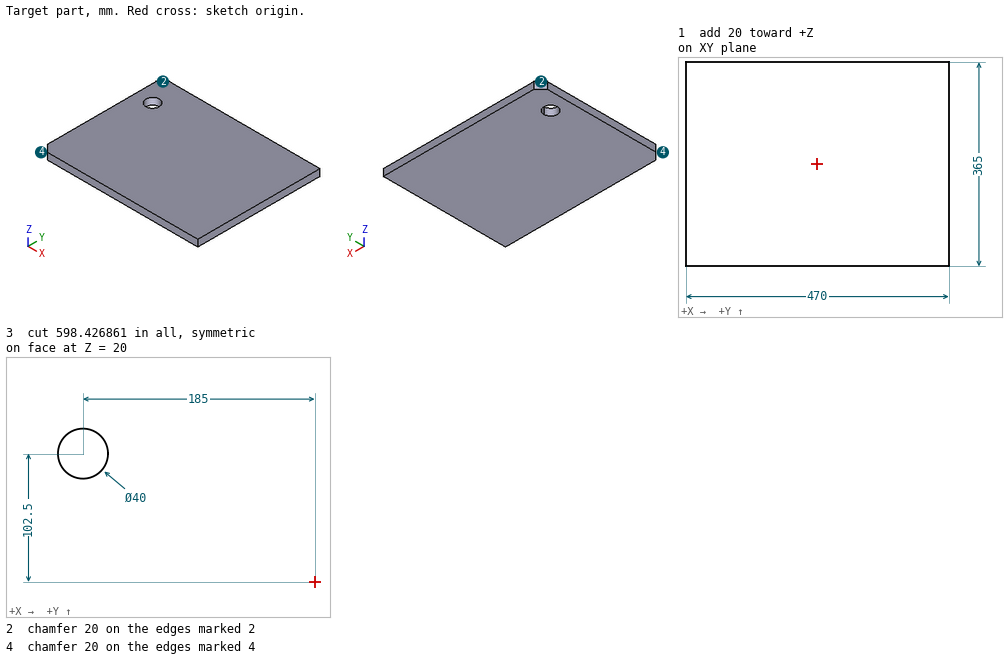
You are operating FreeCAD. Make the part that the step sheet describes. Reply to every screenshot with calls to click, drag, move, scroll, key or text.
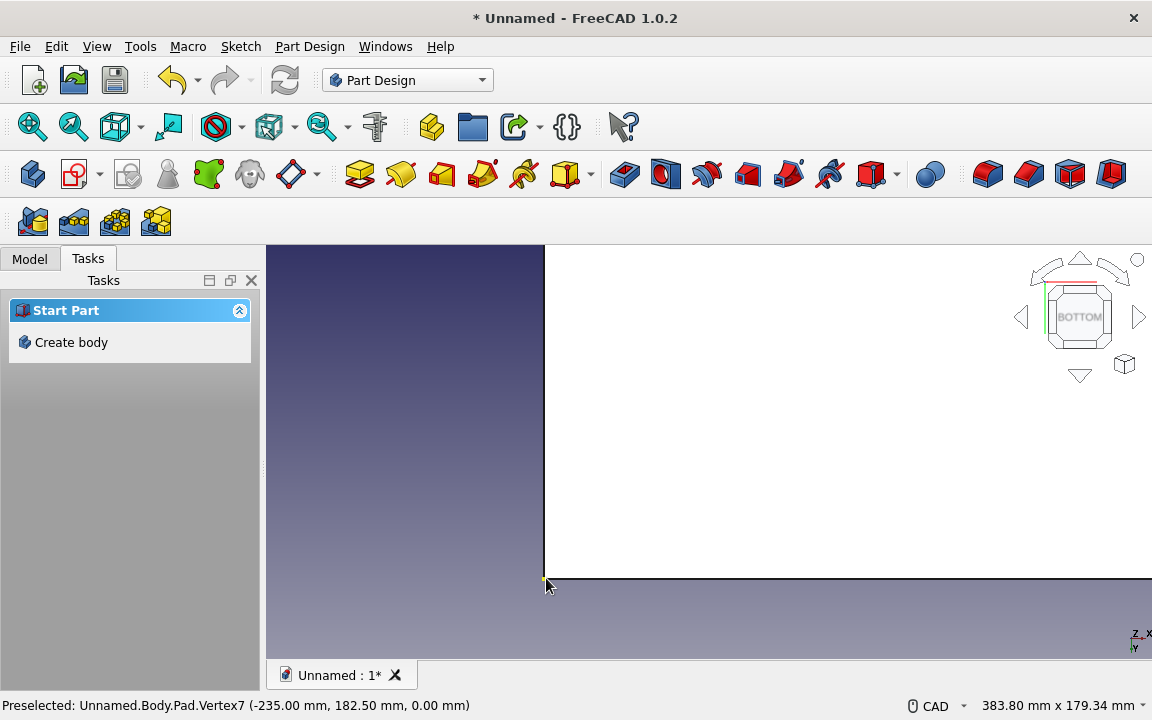
click(33, 128)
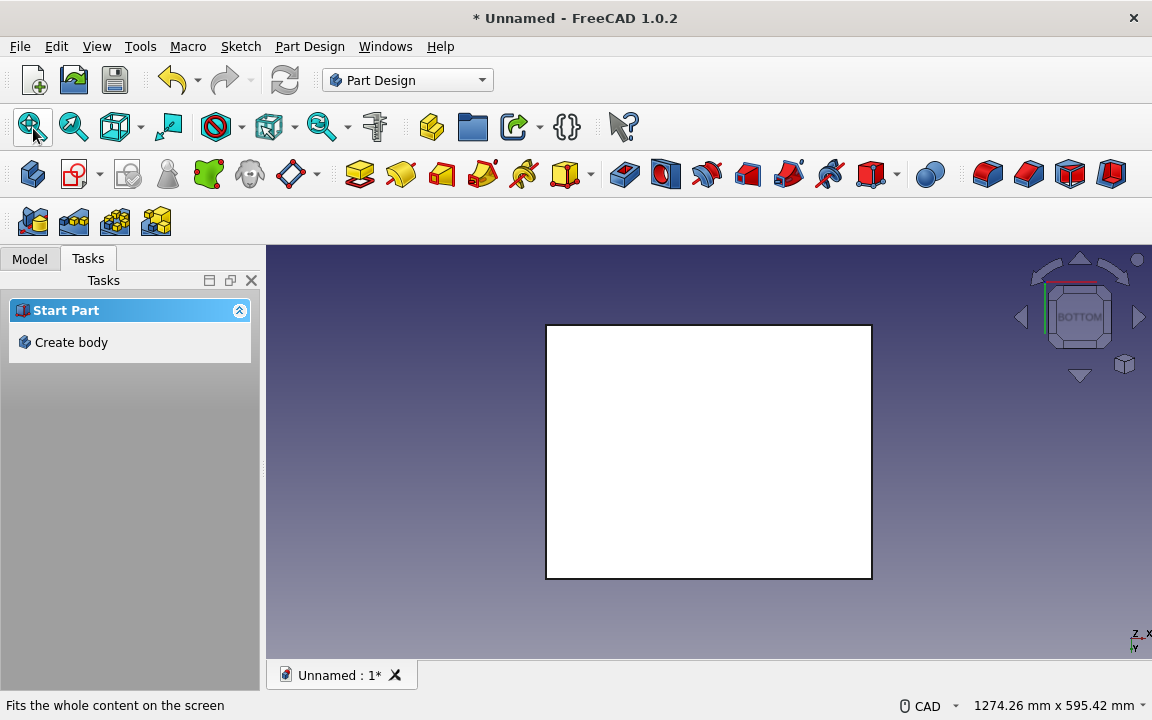
key(4)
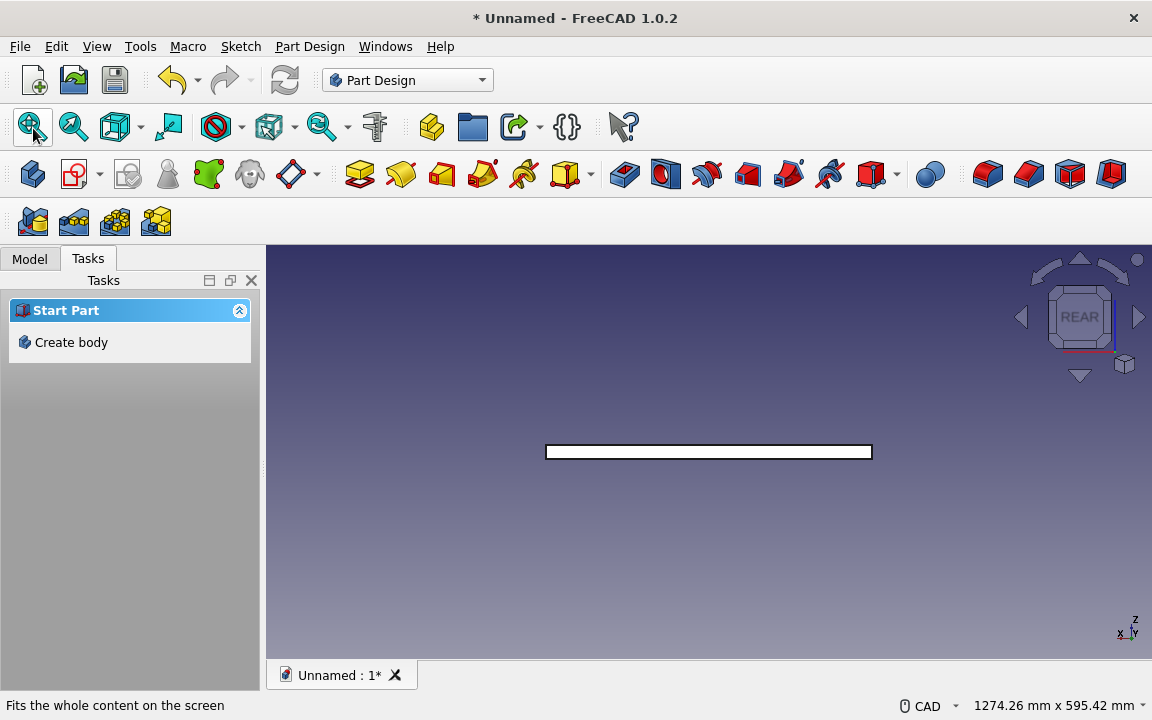
click(33, 128)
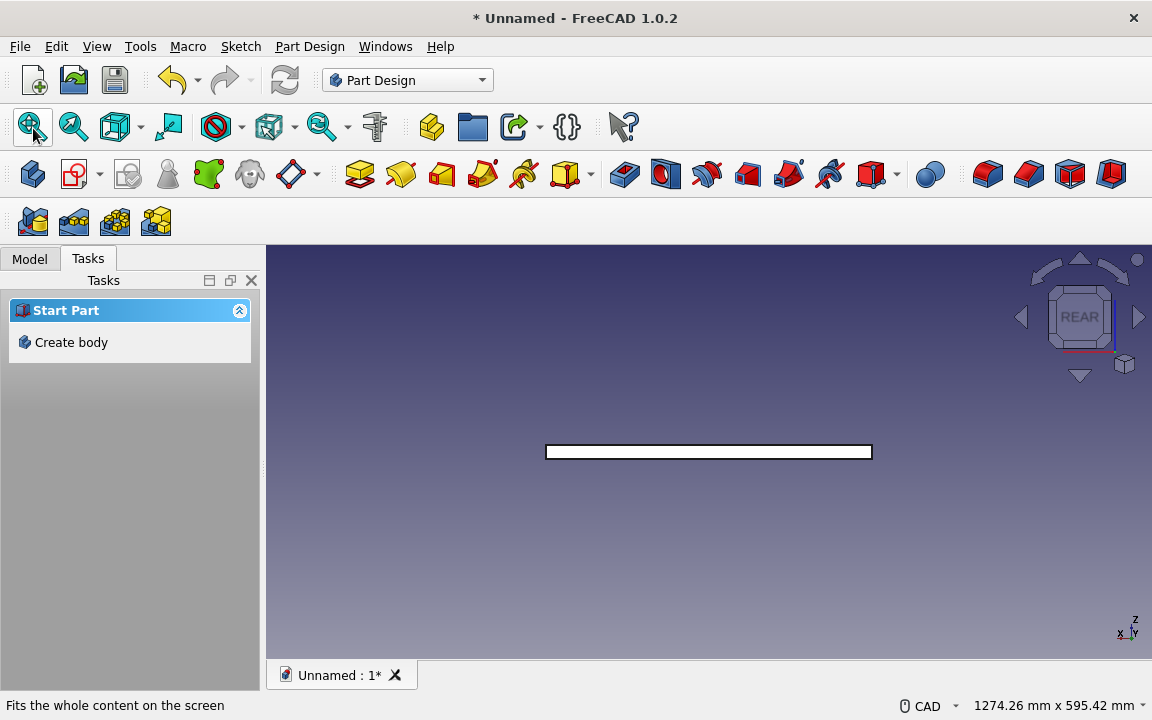
click(872, 451)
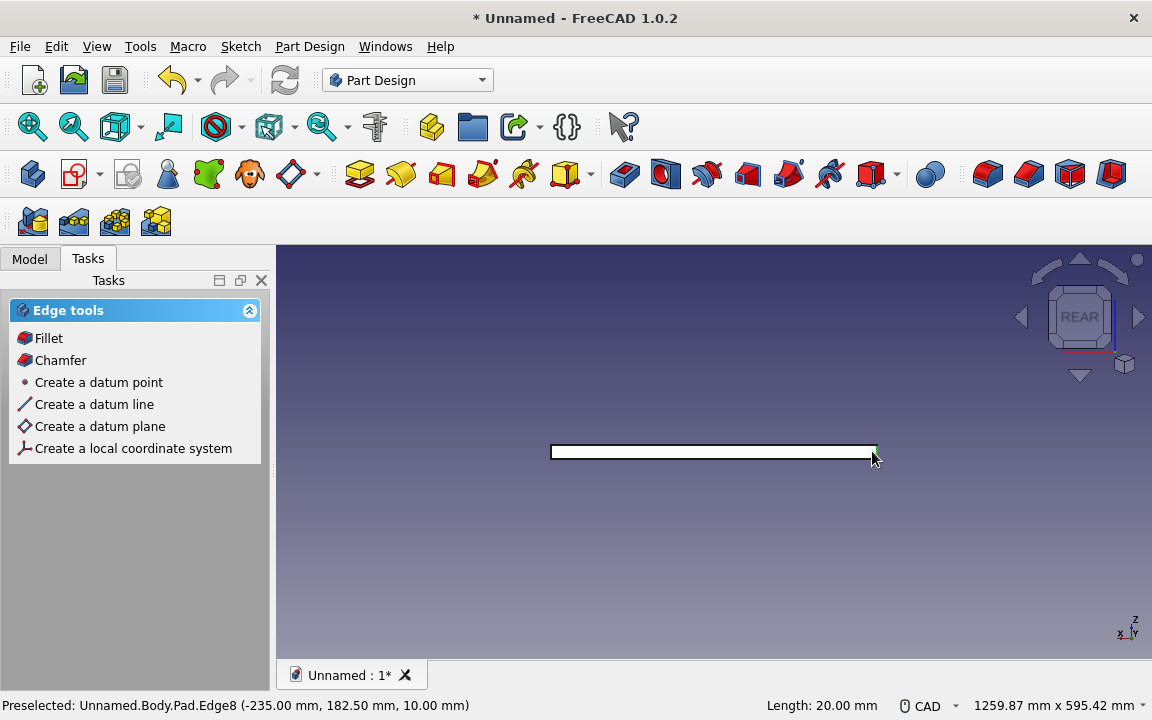
click(1029, 174)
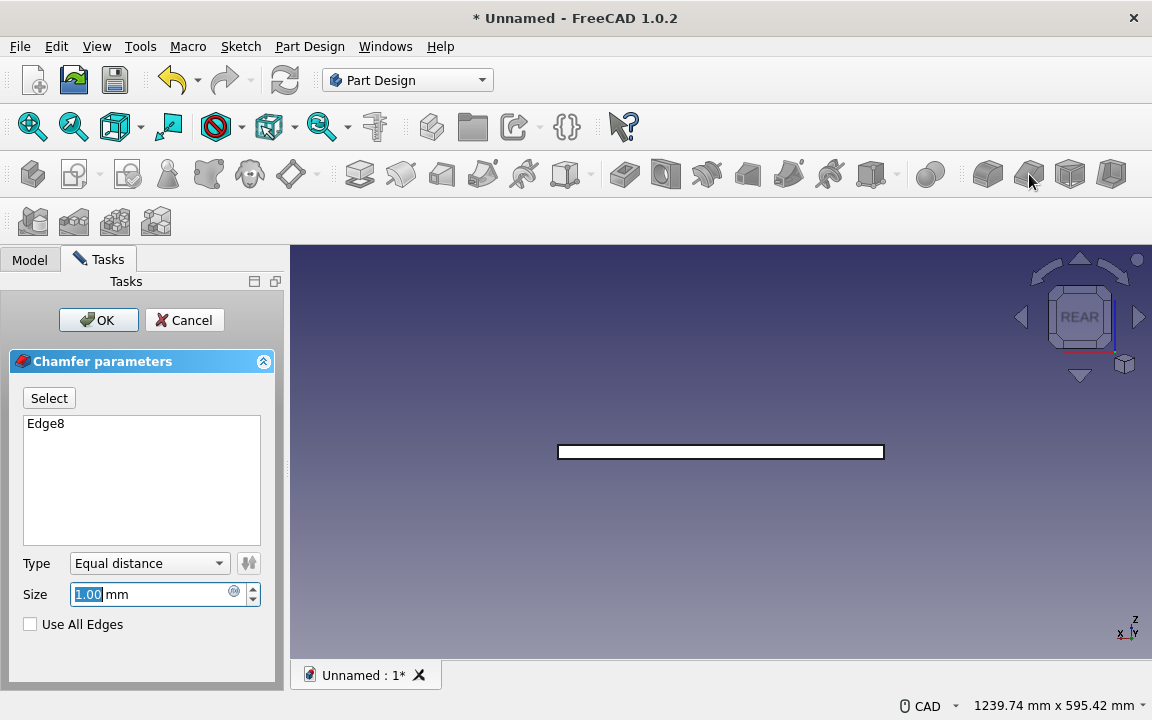
text(20)
key(Tab)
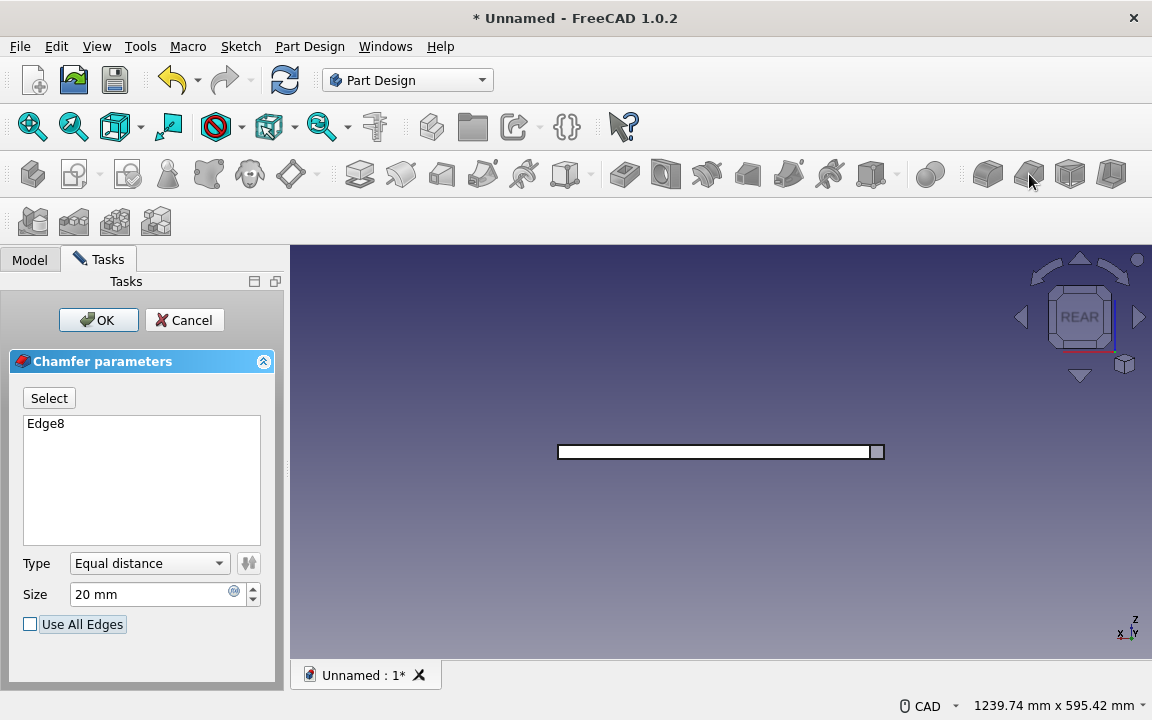
click(99, 320)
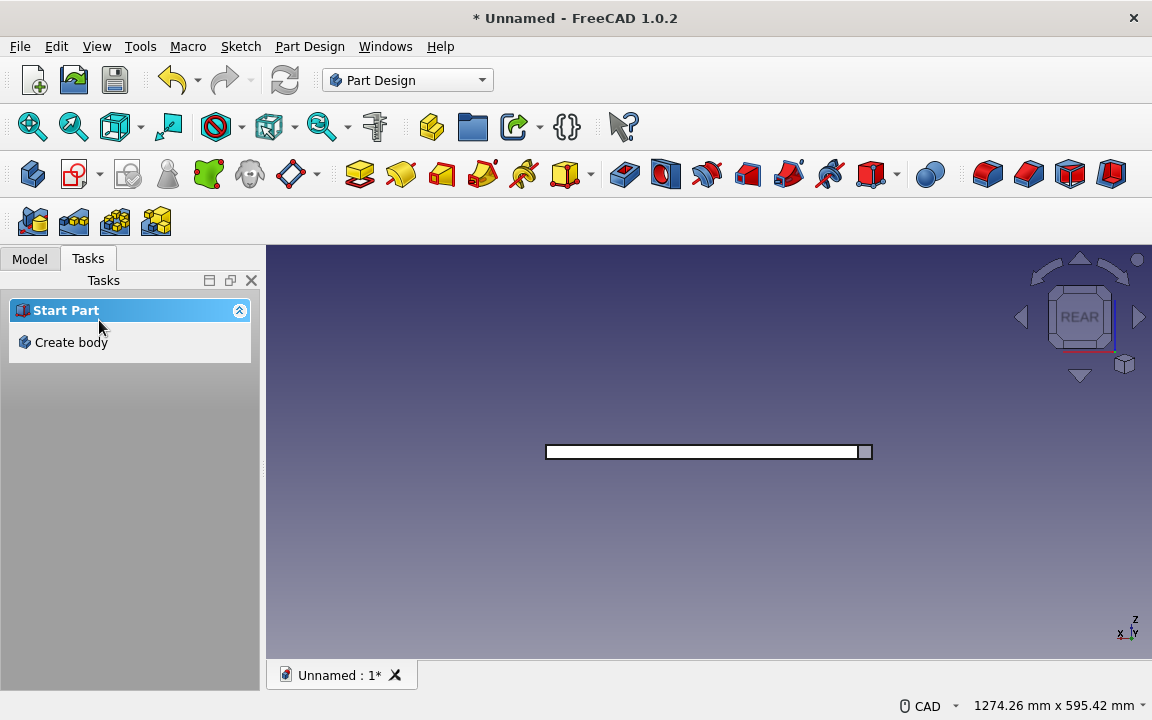
click(33, 128)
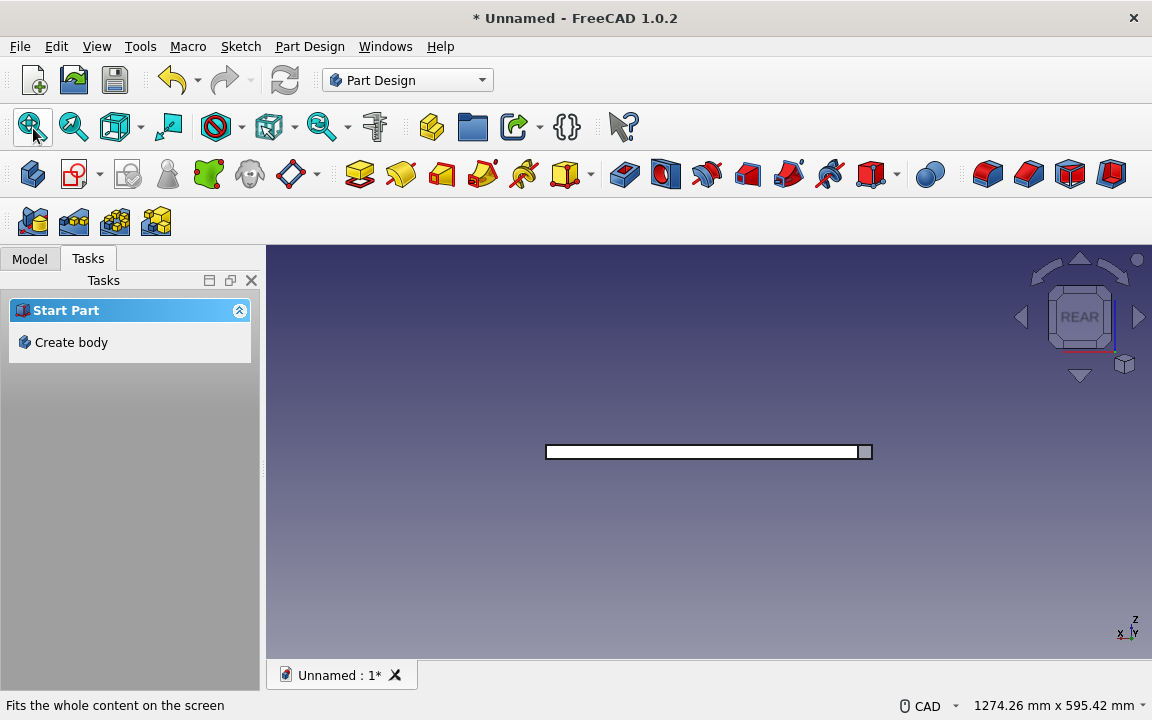
key(0)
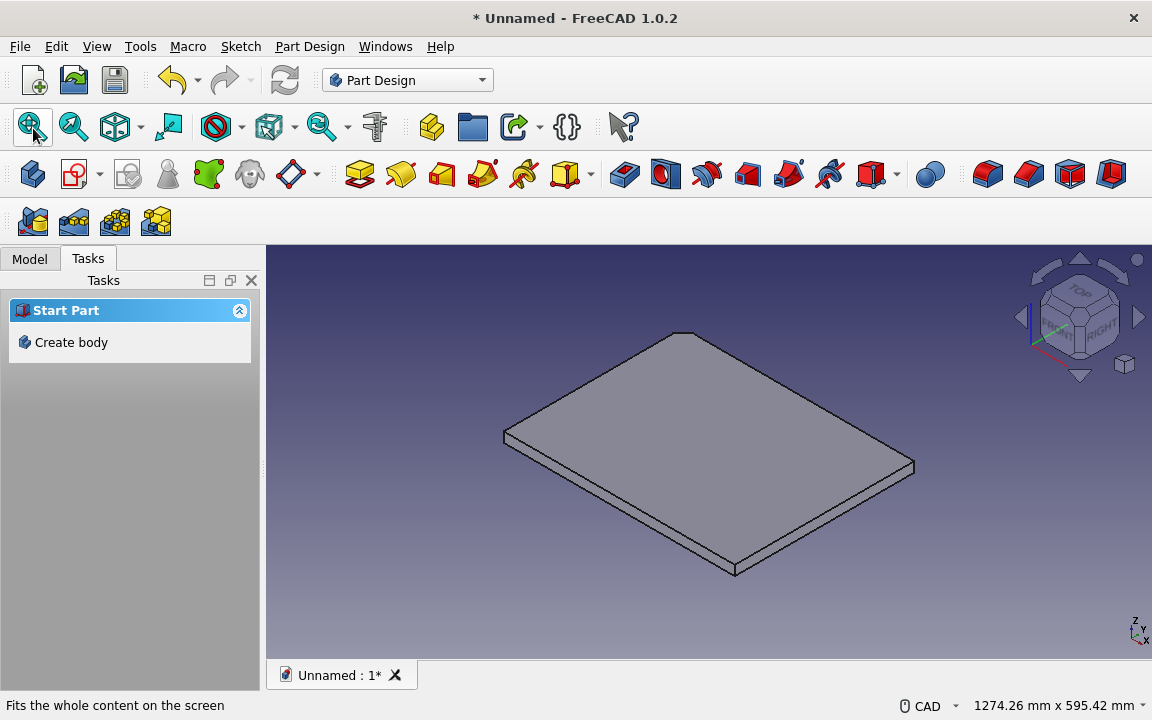
click(709, 445)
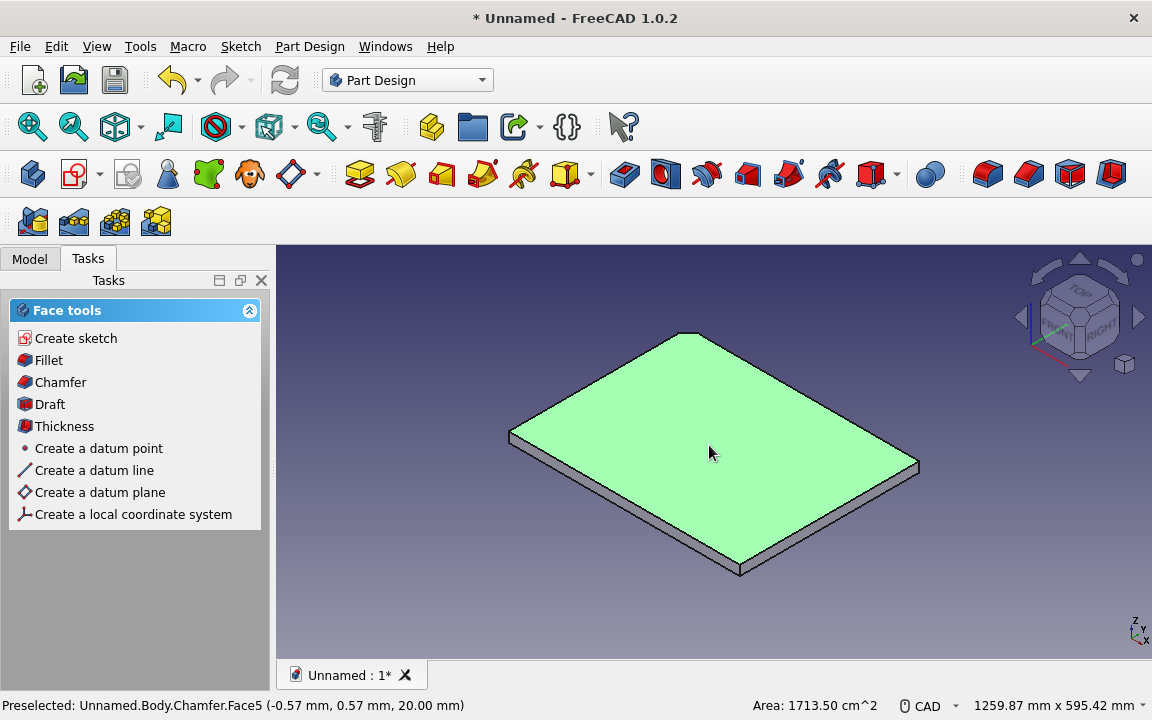
click(74, 174)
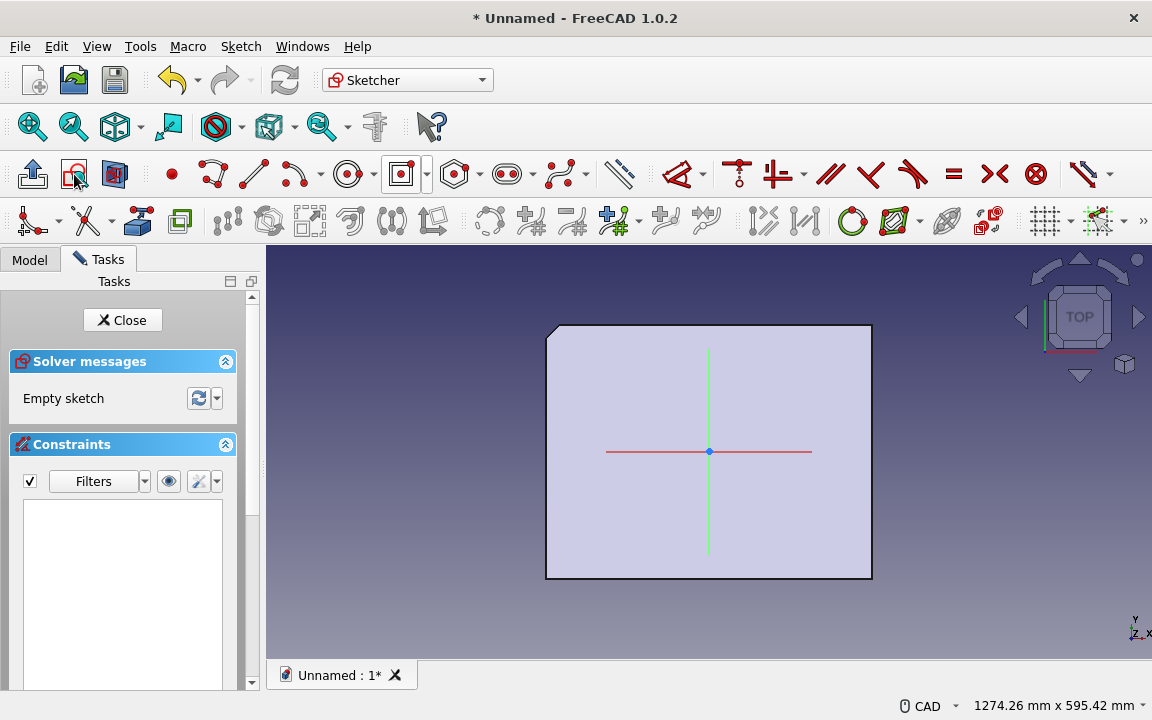
scroll(573, 372, up, 11)